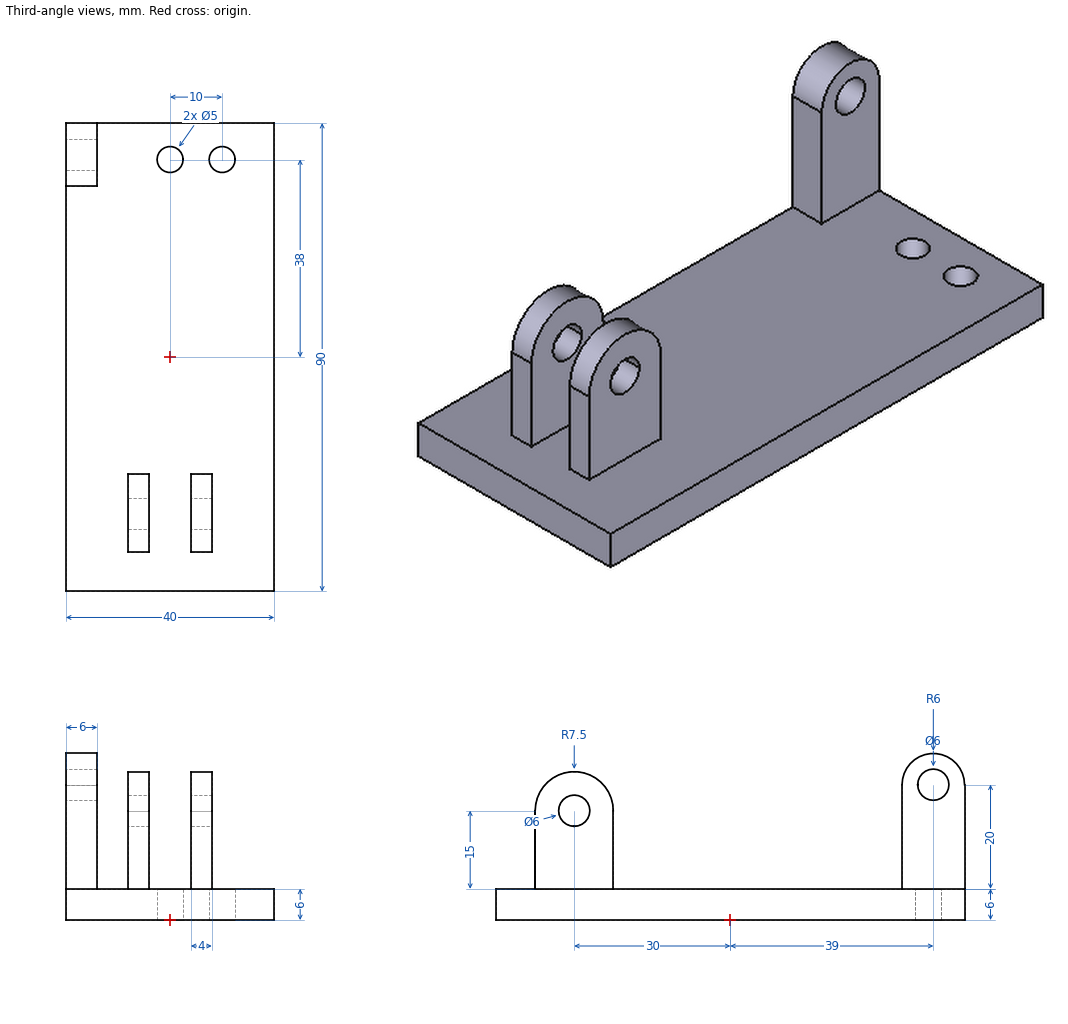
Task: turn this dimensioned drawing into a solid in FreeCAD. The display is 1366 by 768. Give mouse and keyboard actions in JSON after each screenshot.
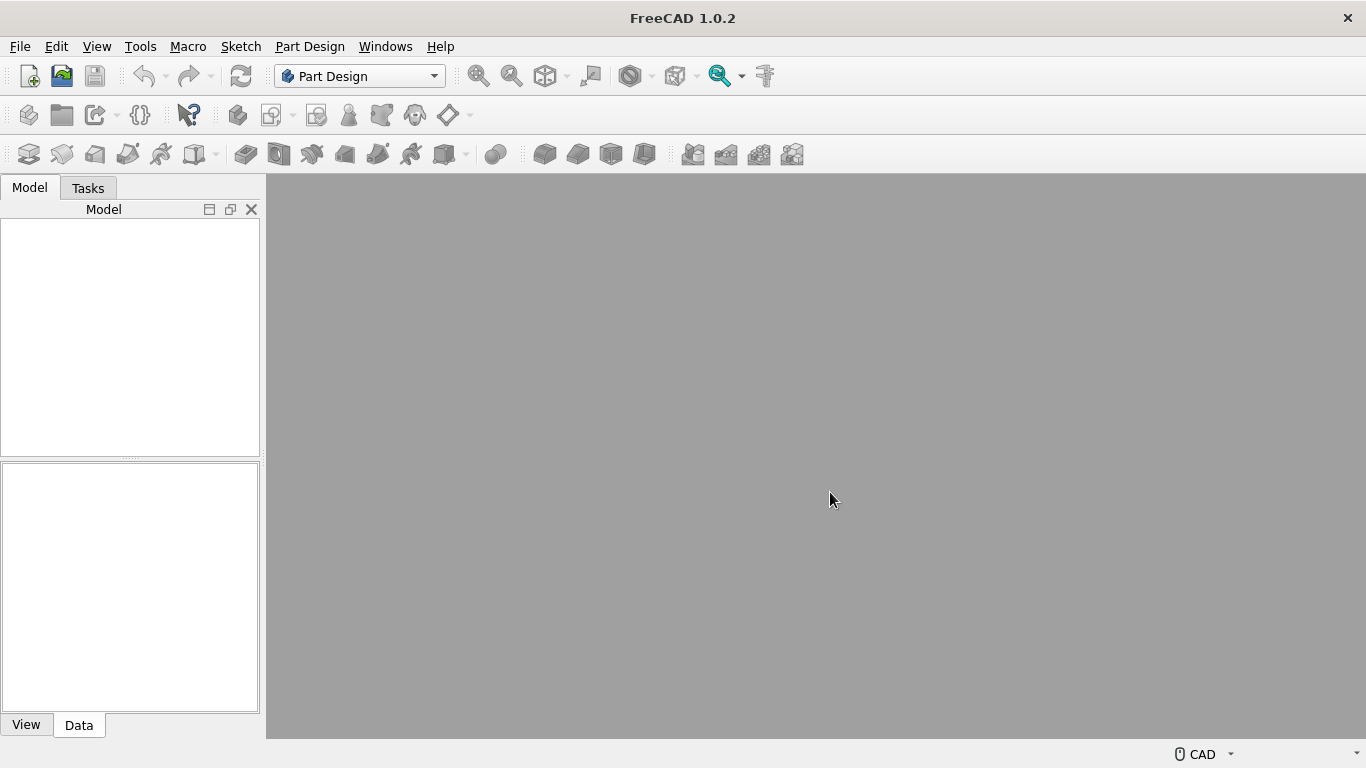
{"action": "key", "text": "ctrl+n"}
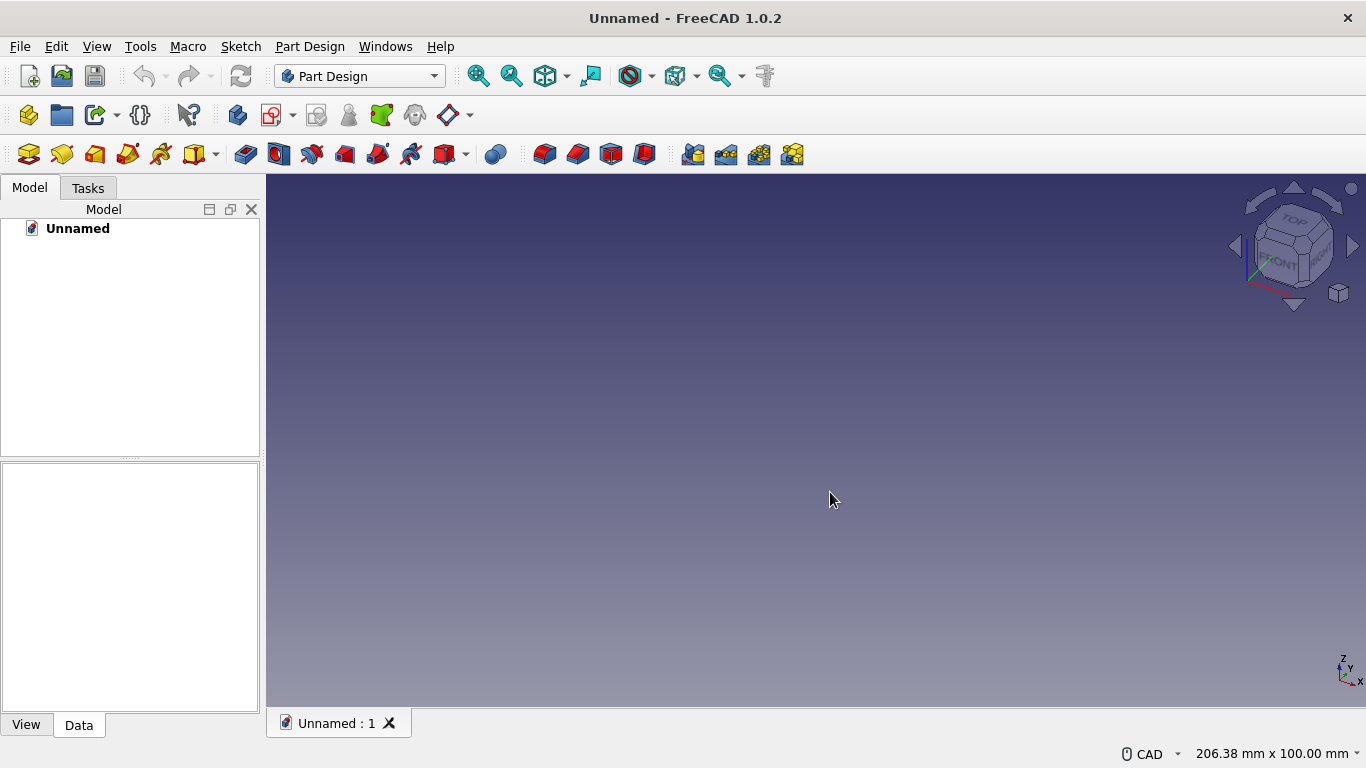
{"action": "left_click", "coordinate": [270, 116]}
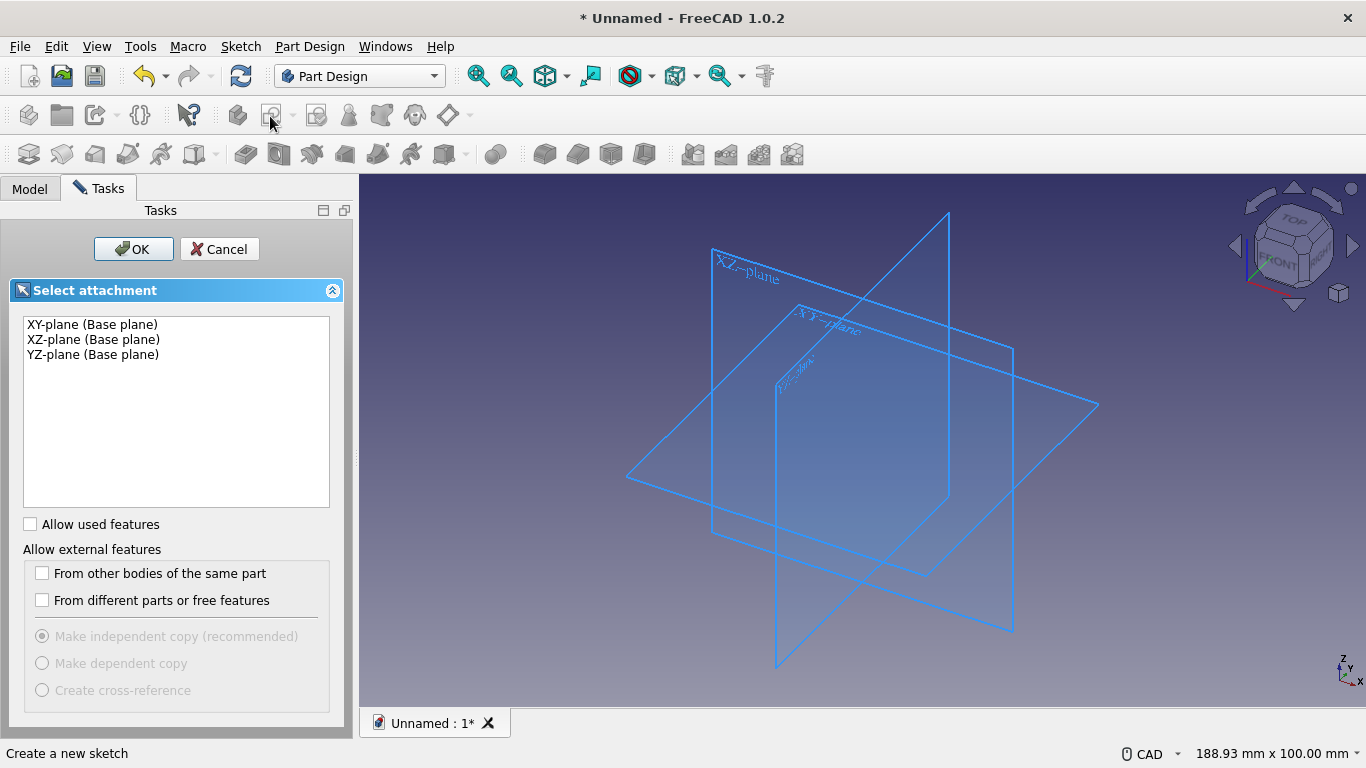
{"action": "left_click", "coordinate": [84, 324]}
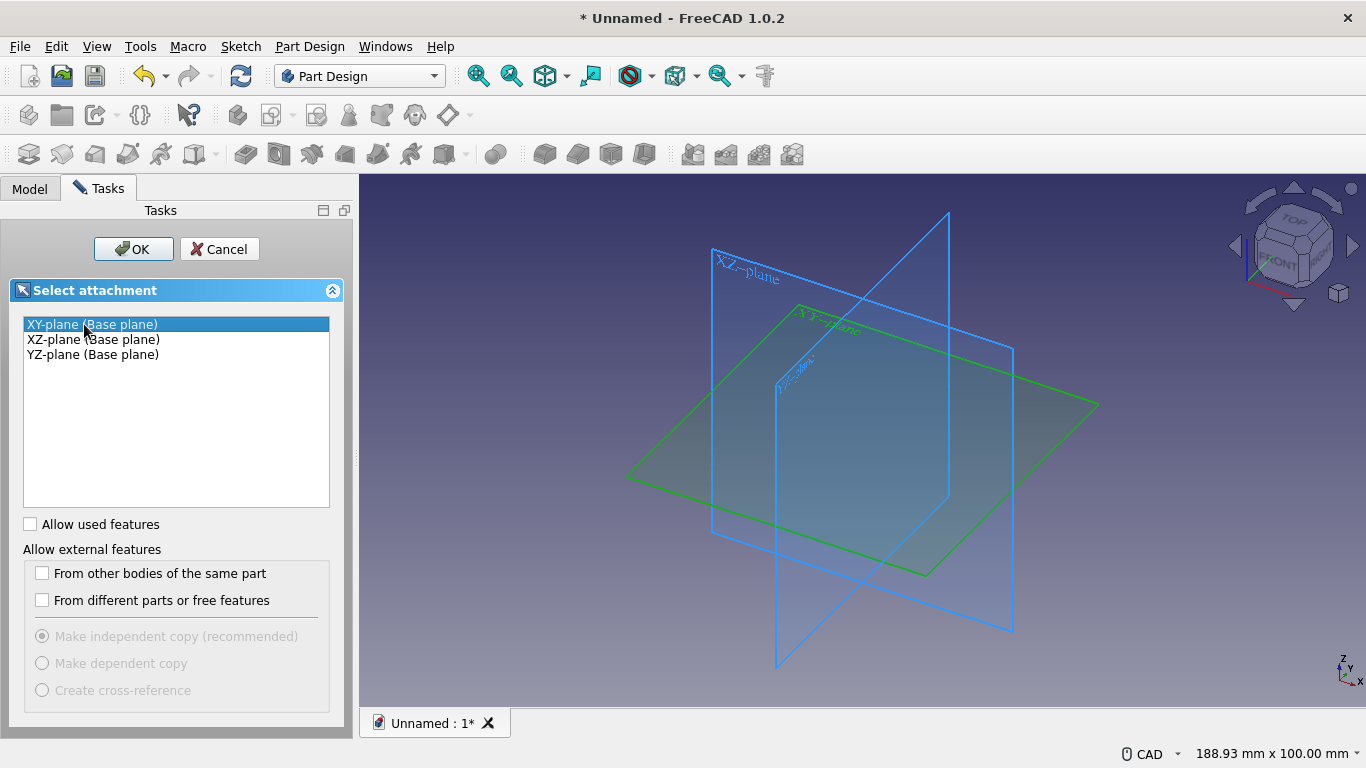
{"action": "left_click", "coordinate": [134, 249]}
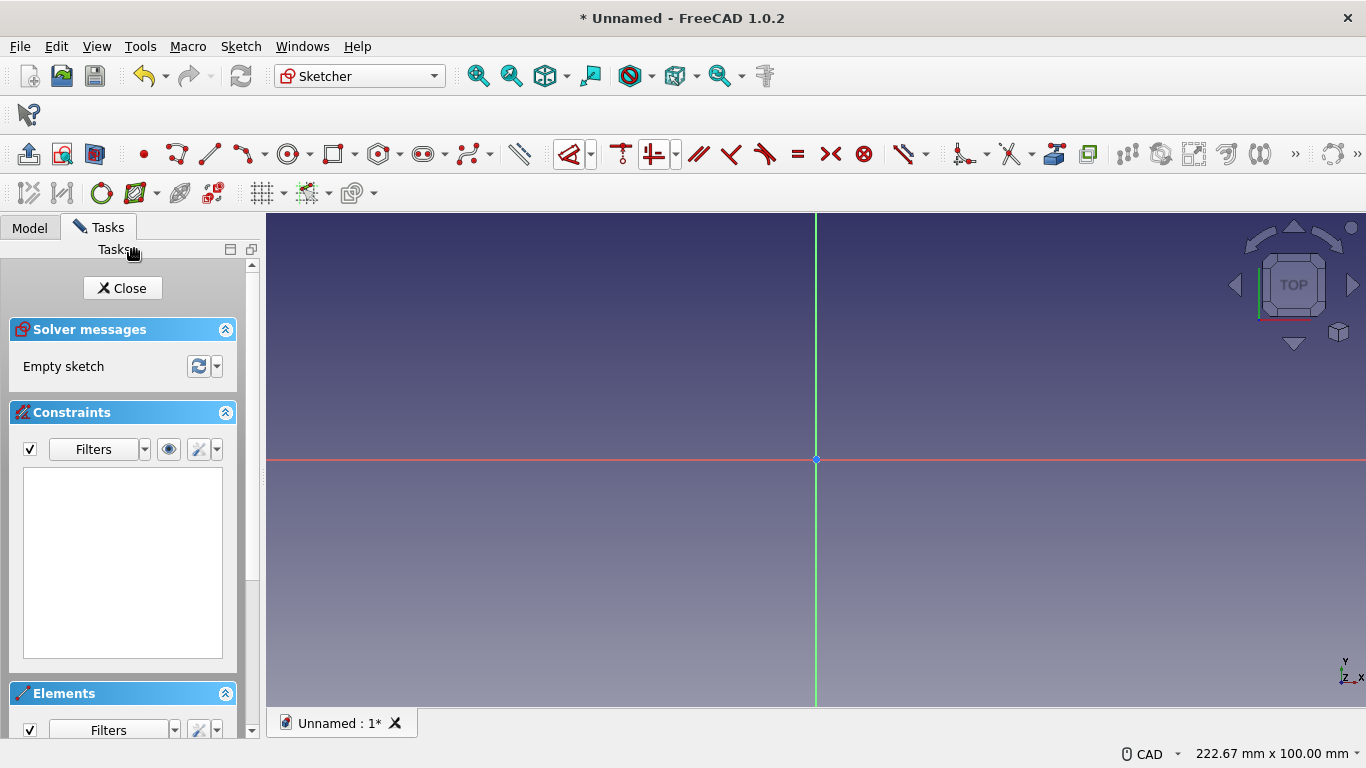
{"action": "scroll", "coordinate": [608, 460], "scroll_direction": "down", "scroll_amount": 2}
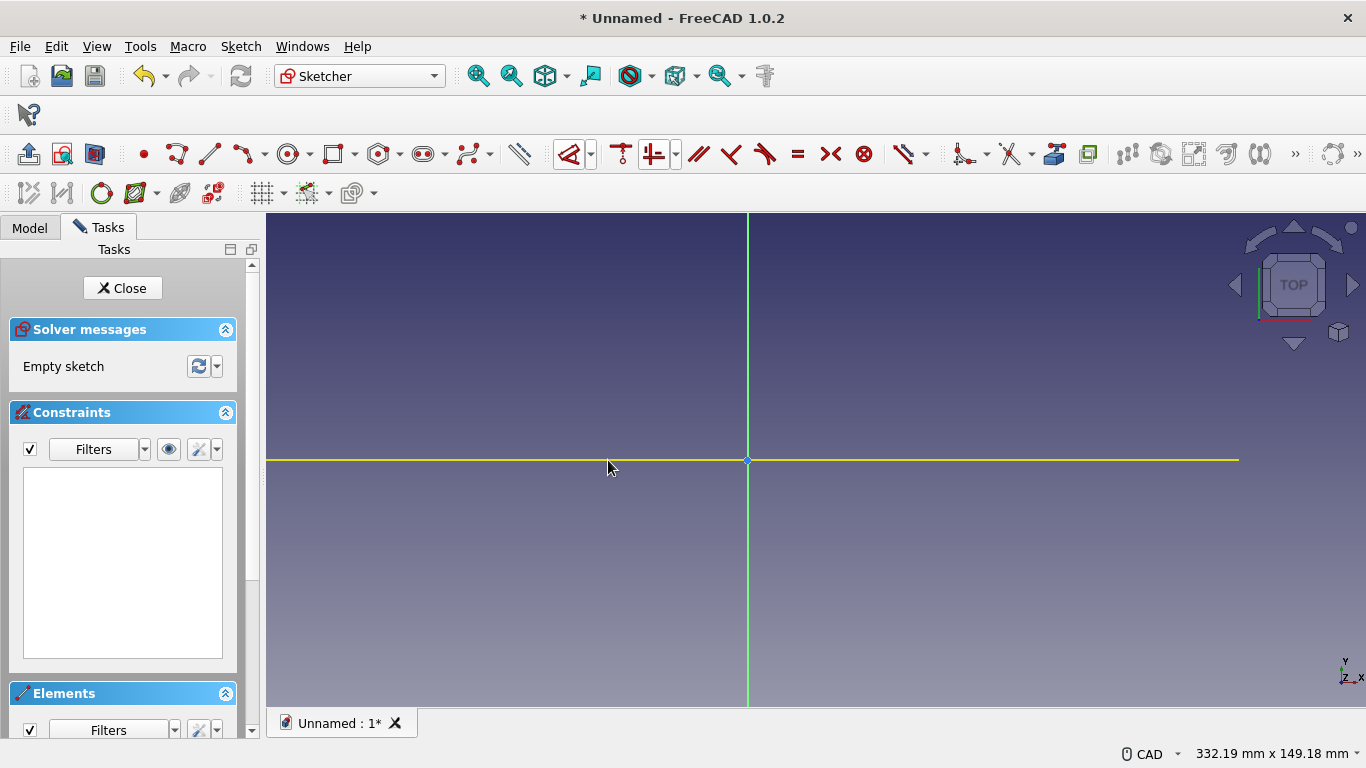
{"action": "key", "text": "g v"}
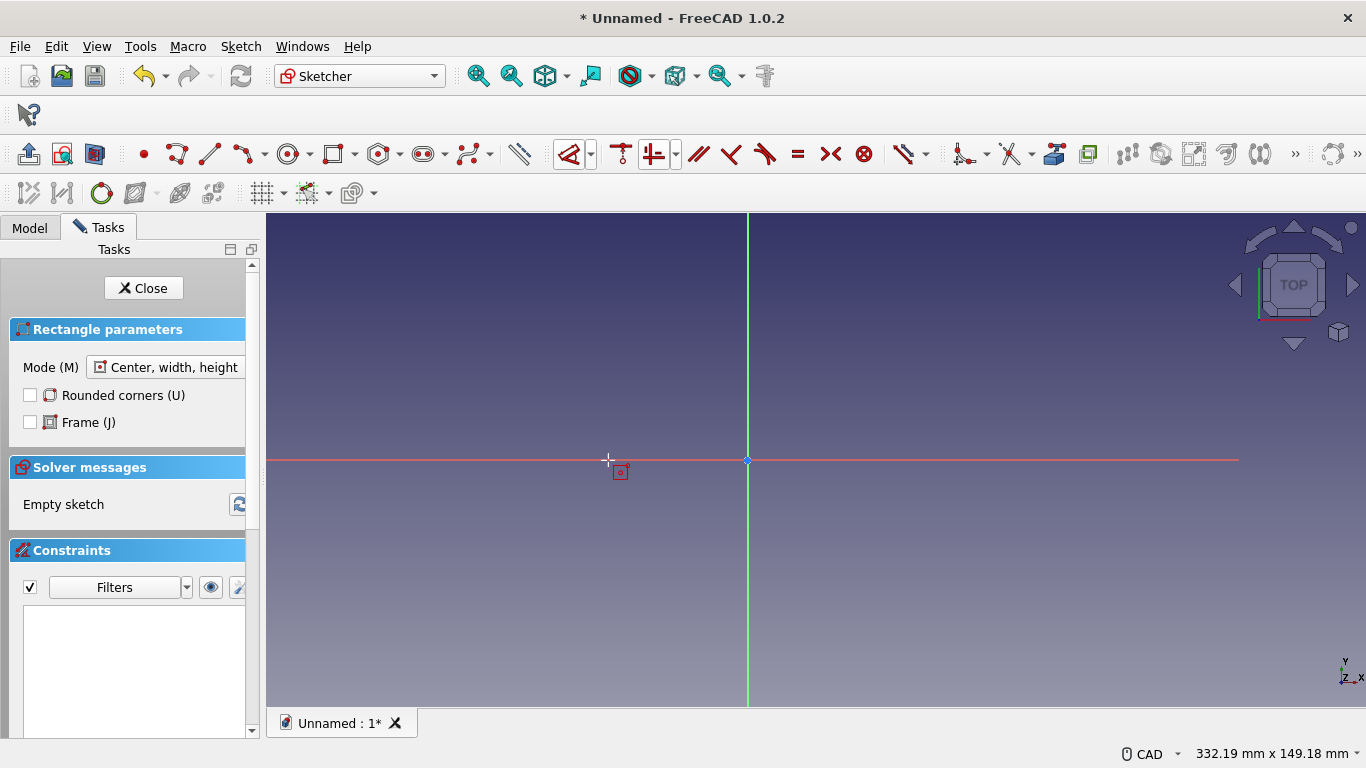
{"action": "left_click", "coordinate": [748, 460]}
{"action": "mouse_move", "coordinate": [814, 311]}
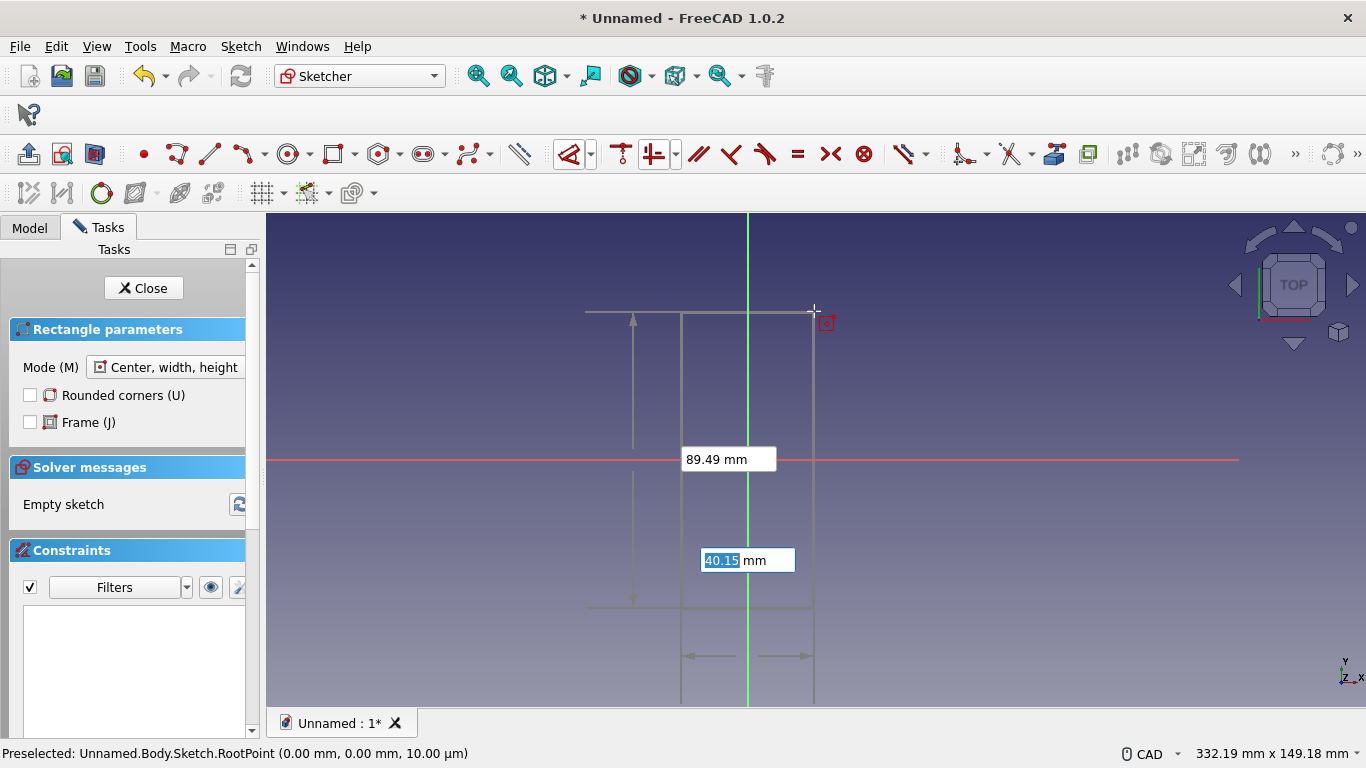
{"action": "type", "text": "40"}
{"action": "key", "text": "Tab"}
{"action": "type", "text": "90"}
{"action": "key", "text": "Return"}
{"action": "key", "text": "Escape"}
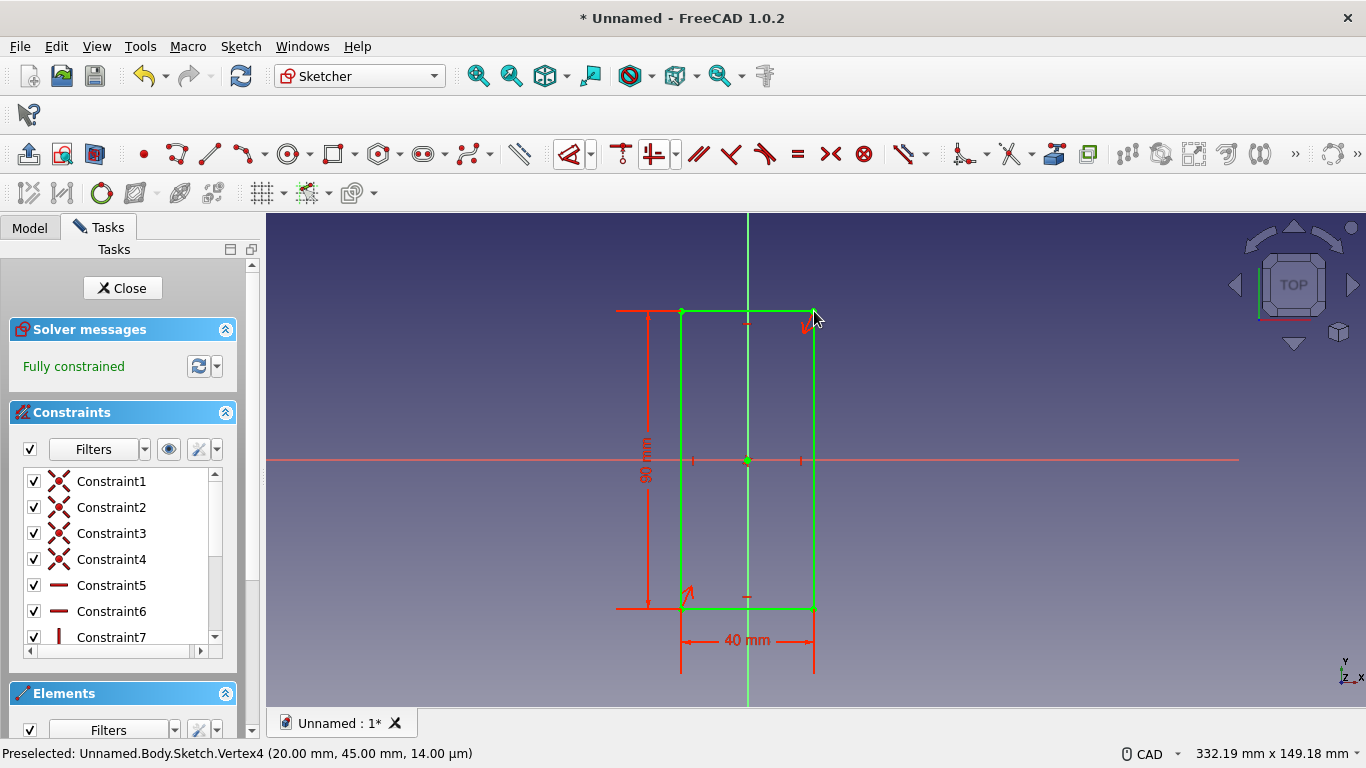
{"action": "left_click", "coordinate": [123, 288]}